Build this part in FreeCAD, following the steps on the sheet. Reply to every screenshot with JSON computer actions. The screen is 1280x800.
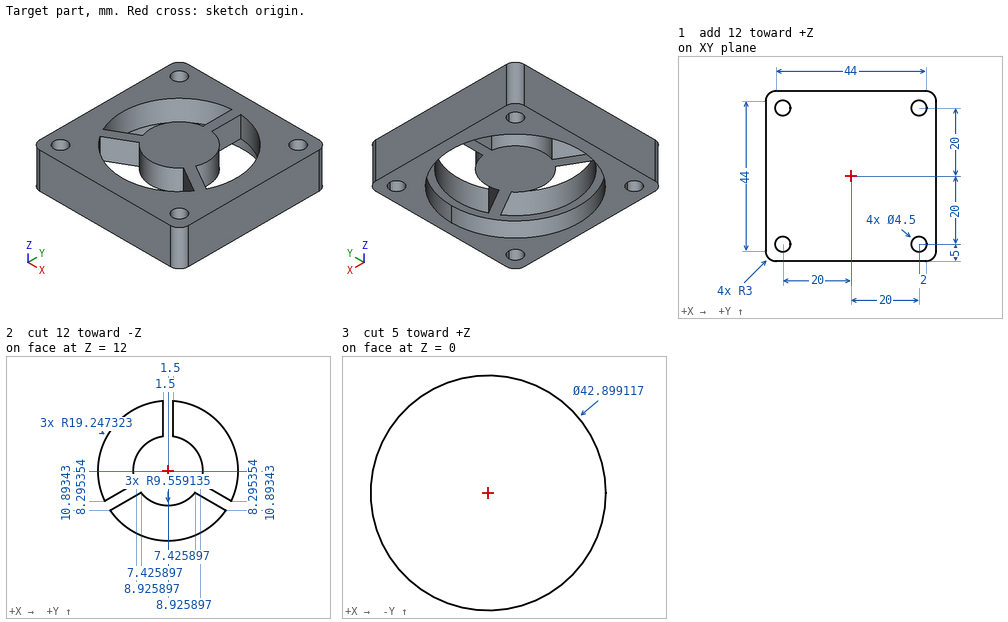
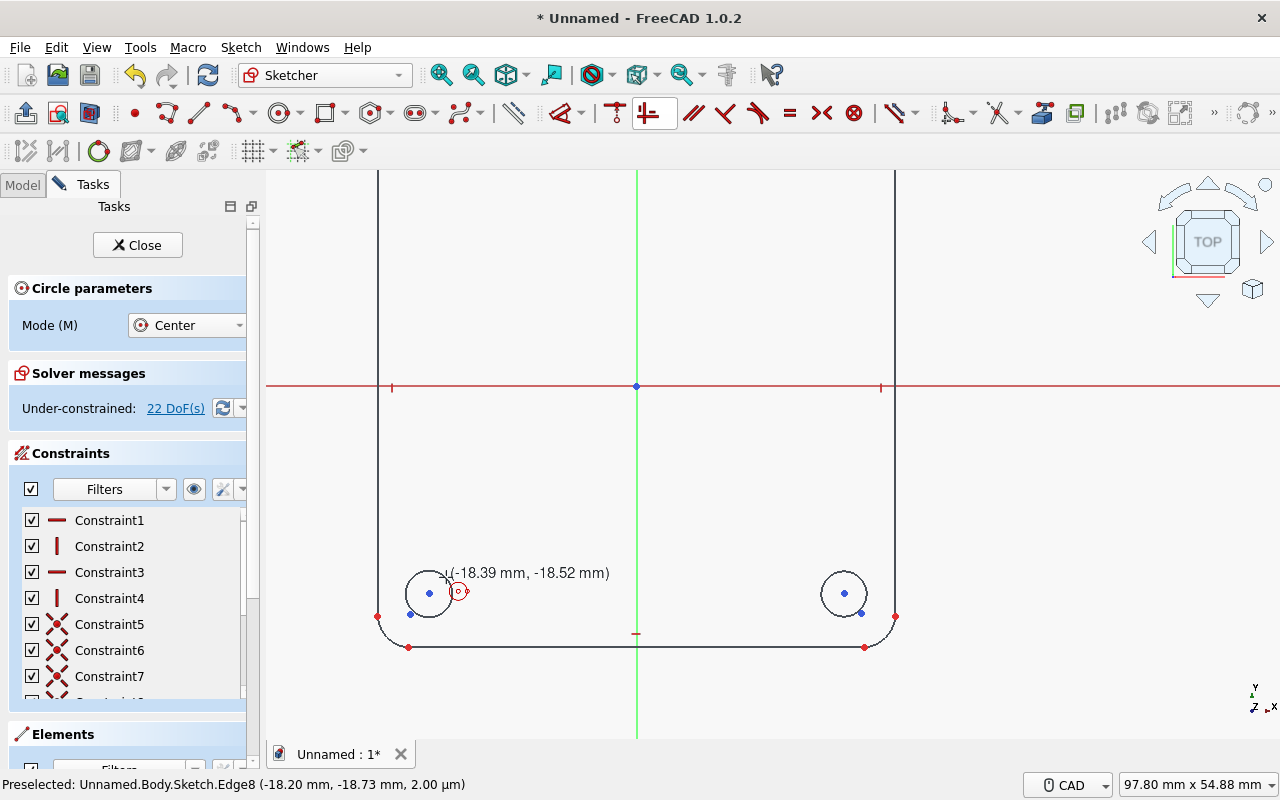
{"action": "scroll", "coordinate": [843, 594], "scroll_direction": "down", "scroll_amount": 2}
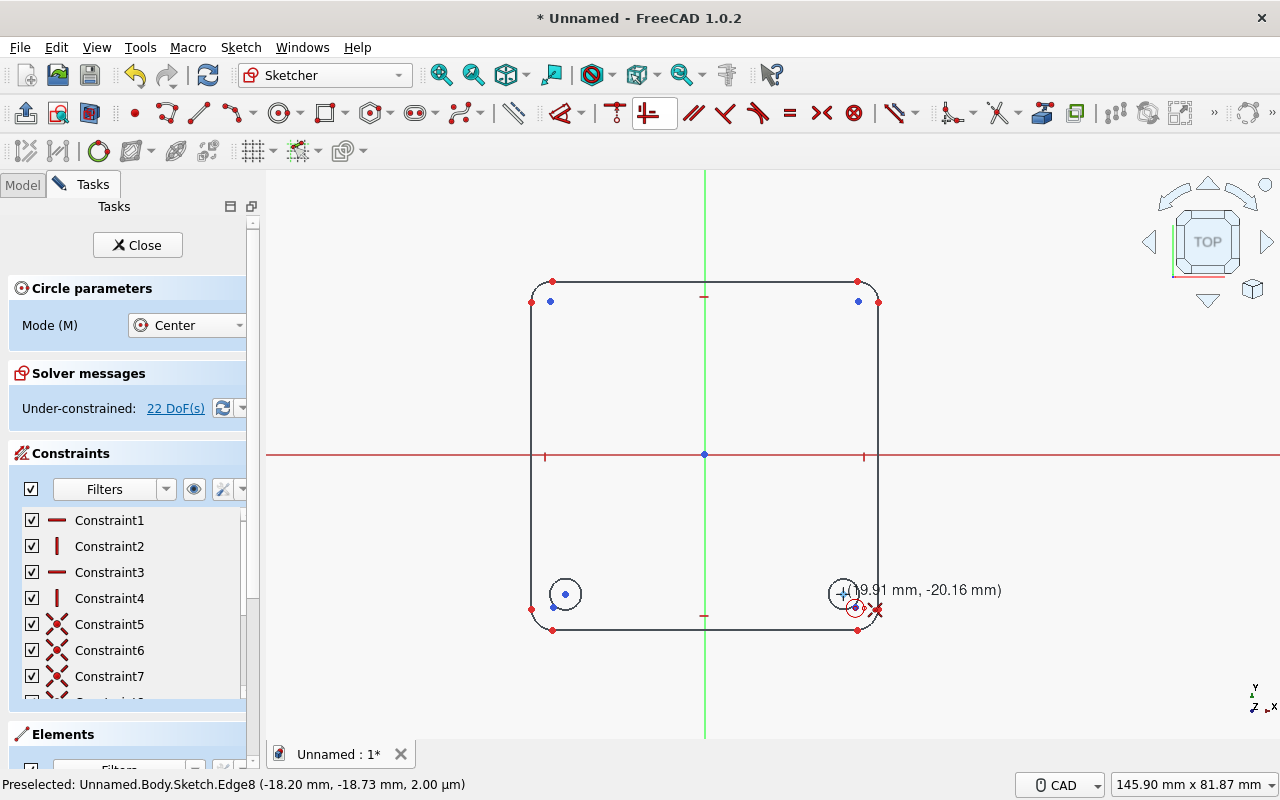
{"action": "scroll", "coordinate": [844, 316], "scroll_direction": "up", "scroll_amount": 2}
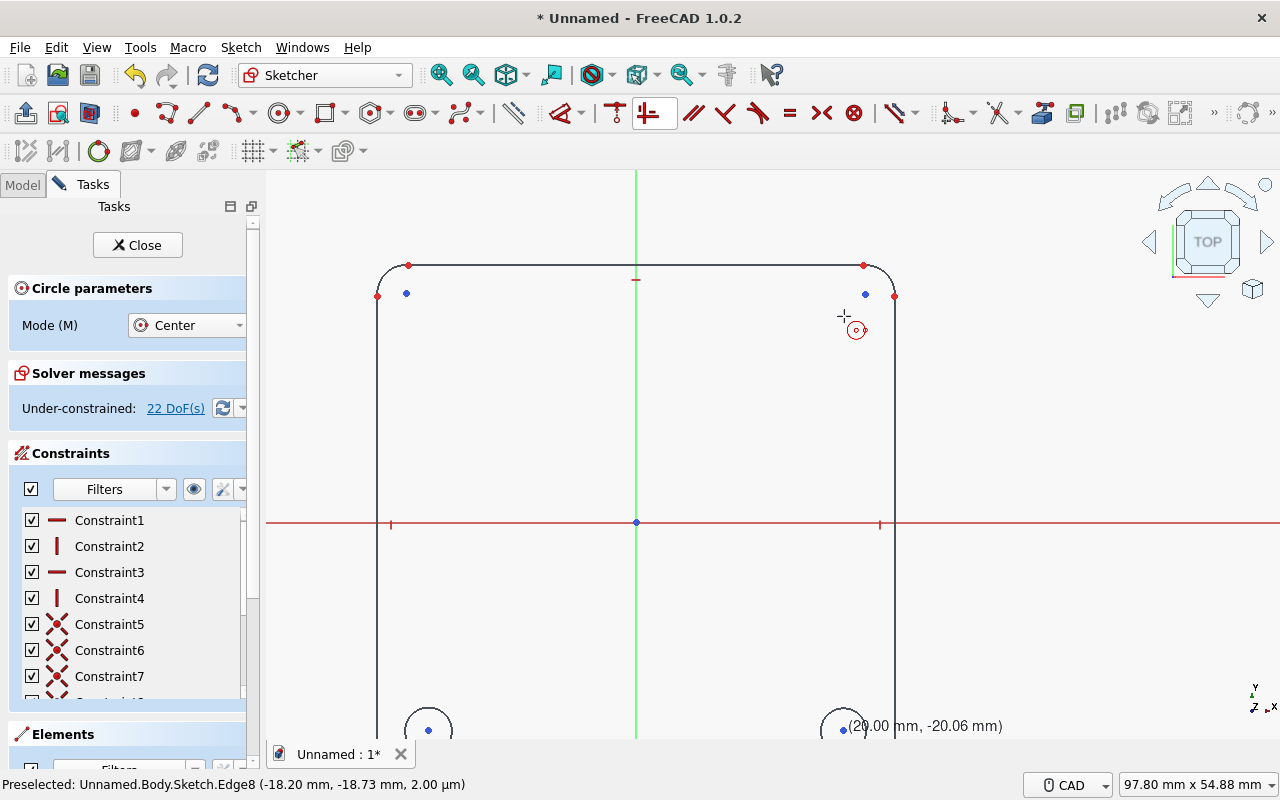
{"action": "left_click", "coordinate": [843, 316]}
{"action": "left_click", "coordinate": [827, 299]}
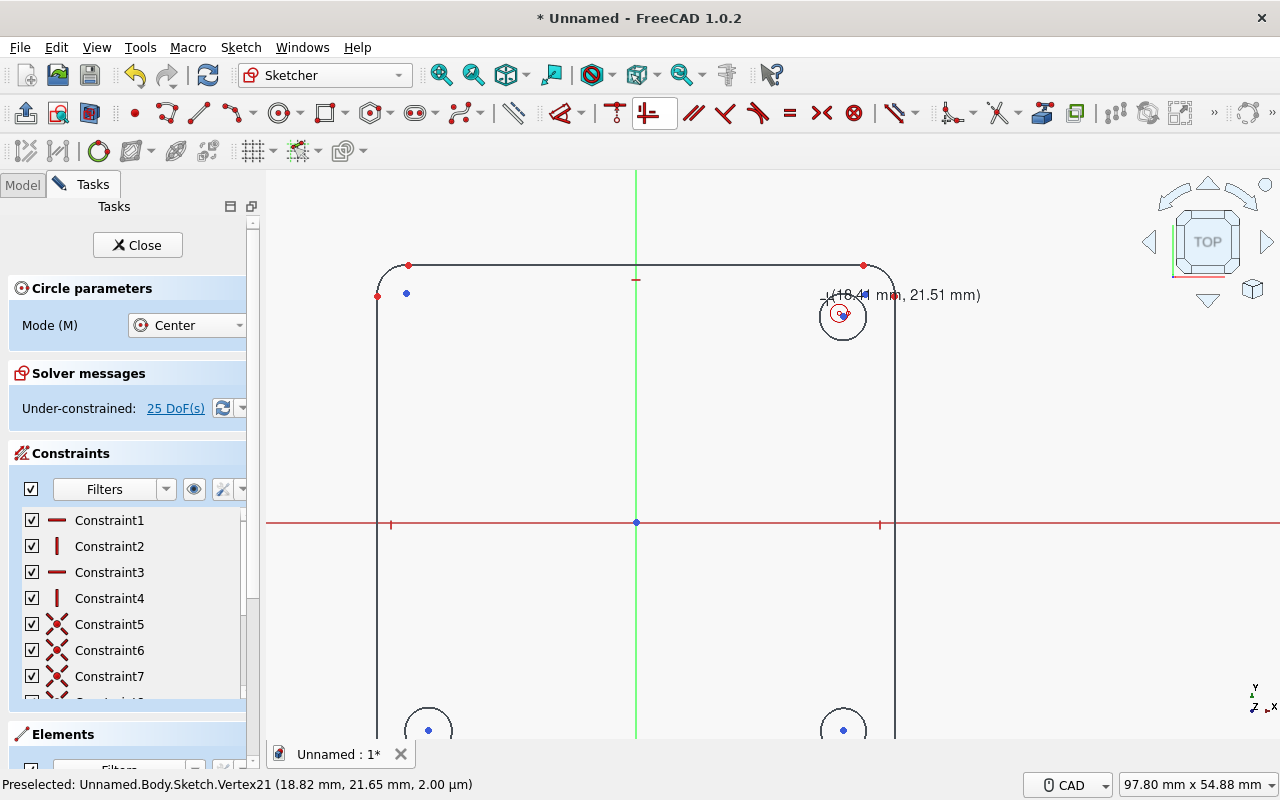
{"action": "left_click", "coordinate": [429, 316]}
{"action": "left_click", "coordinate": [445, 299]}
{"action": "key", "text": "Escape"}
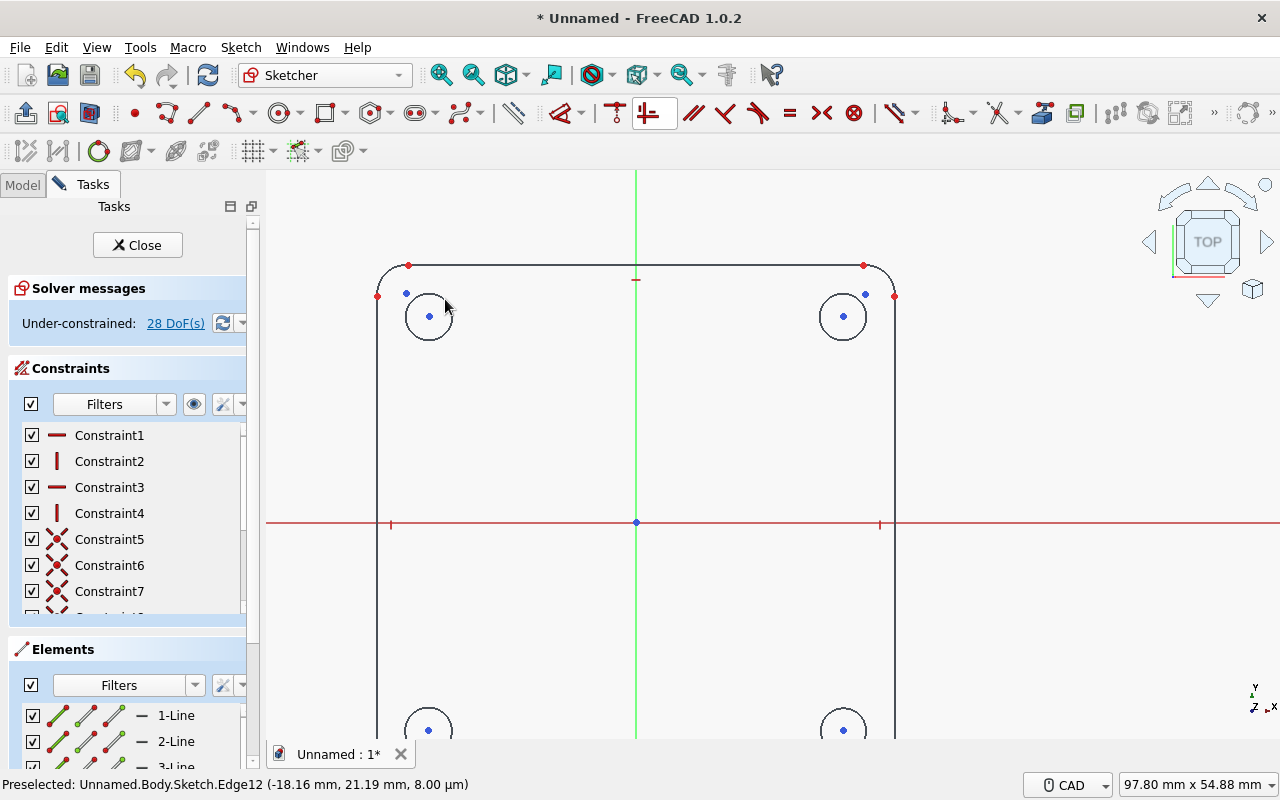
{"action": "left_click", "coordinate": [727, 265]}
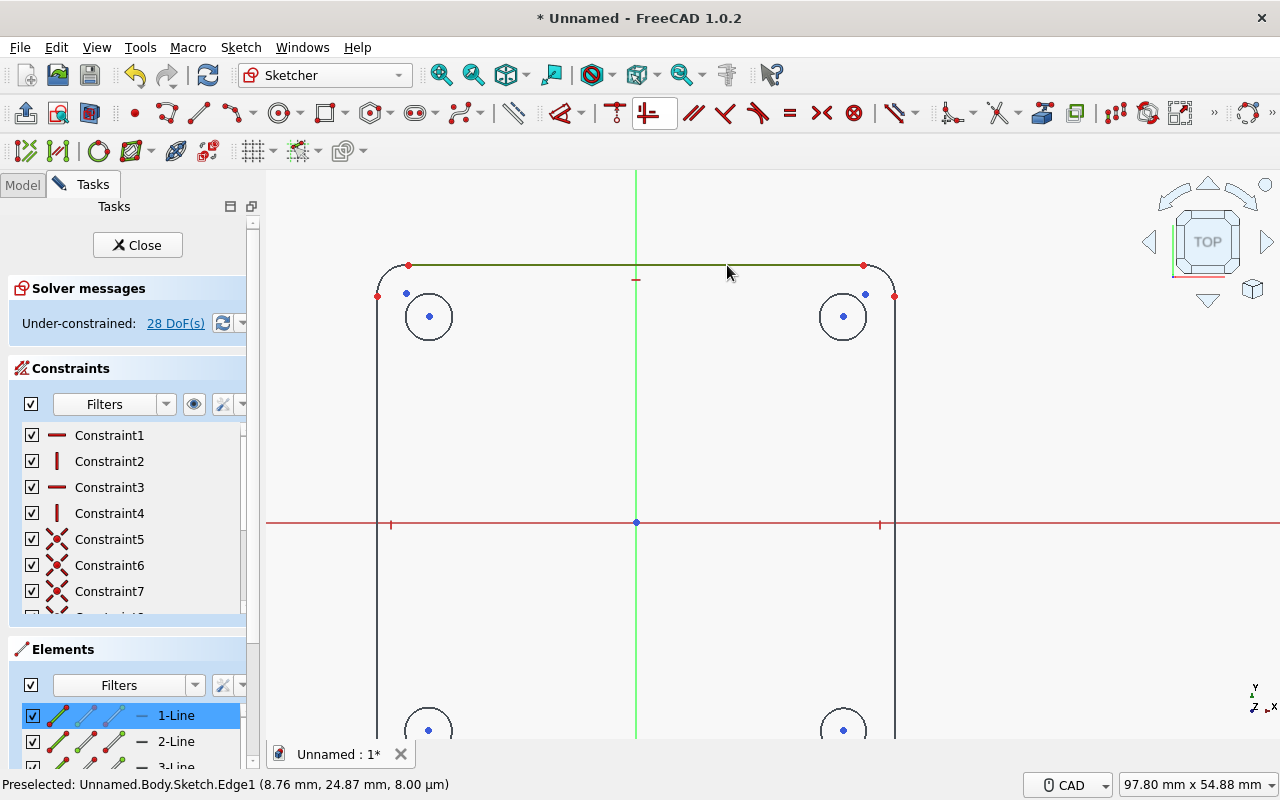
{"action": "left_click", "coordinate": [394, 268]}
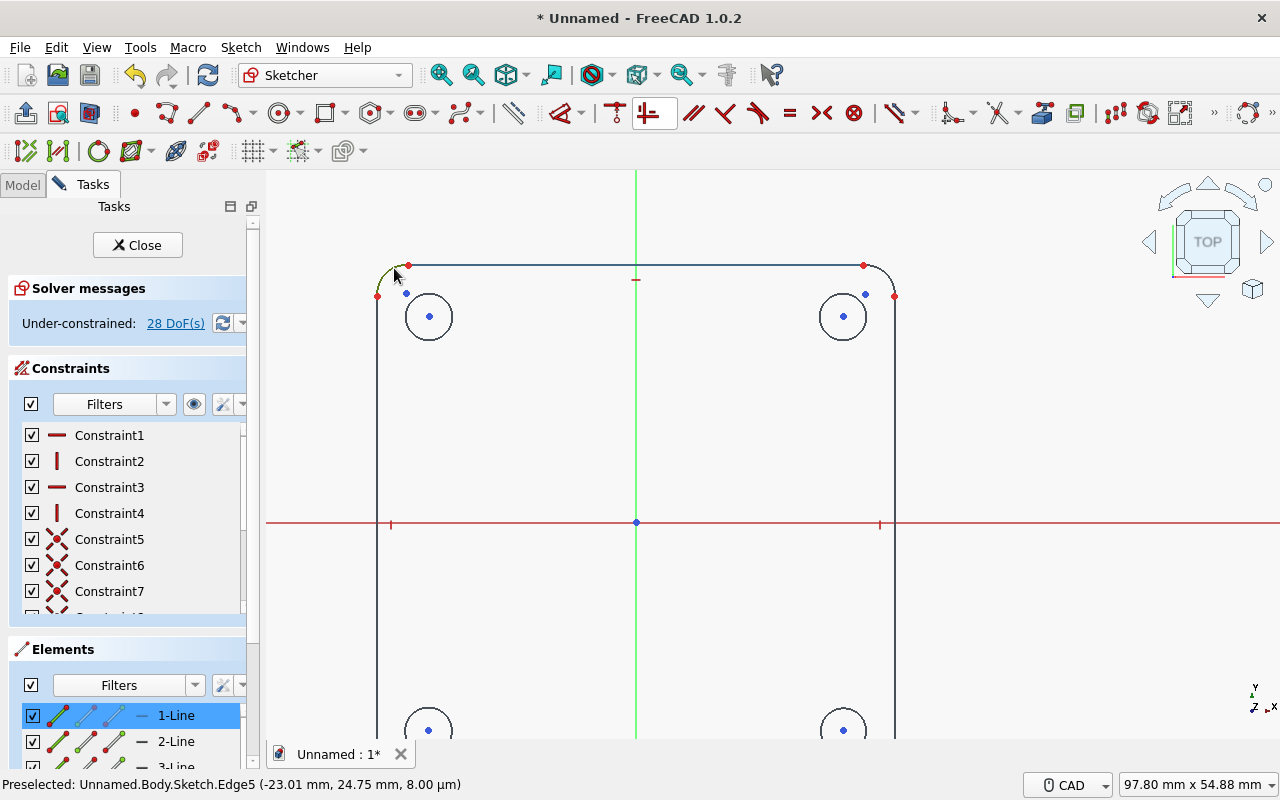
{"action": "left_click", "coordinate": [758, 114]}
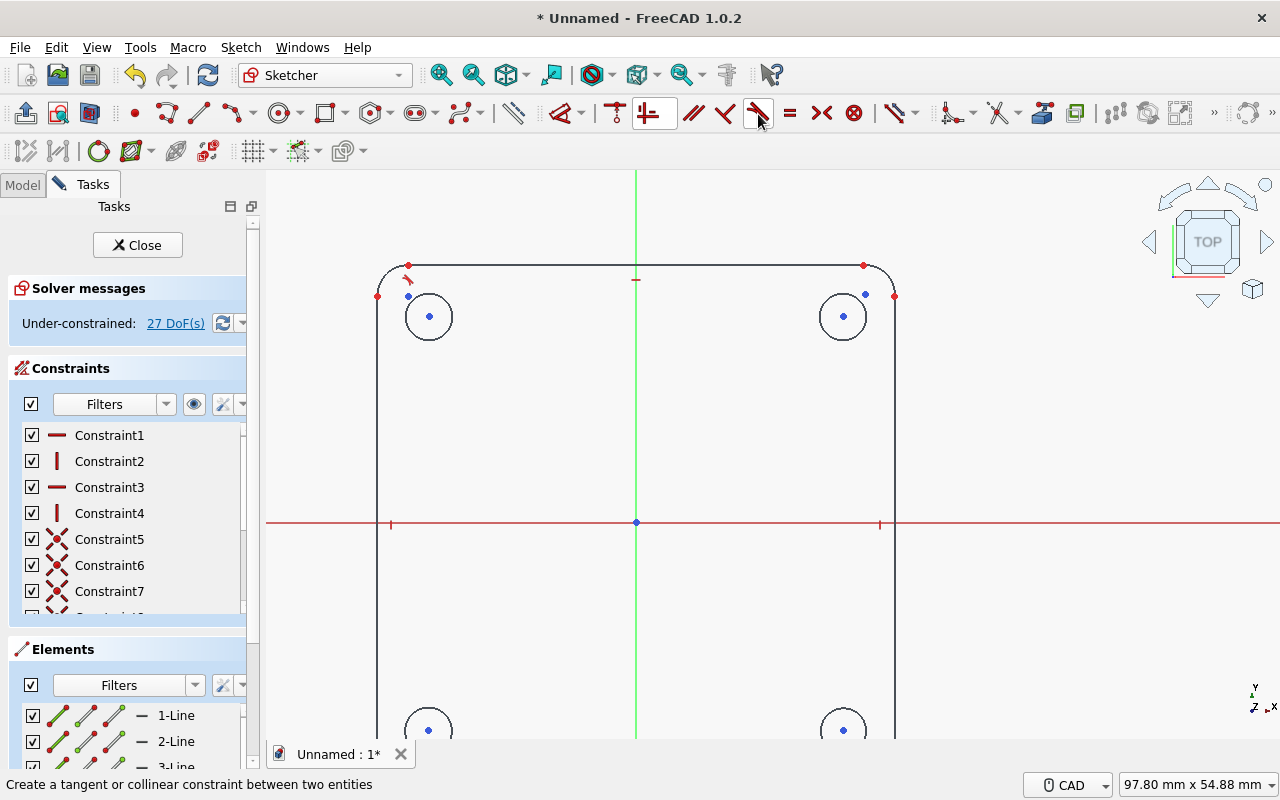
{"action": "left_click", "coordinate": [727, 265]}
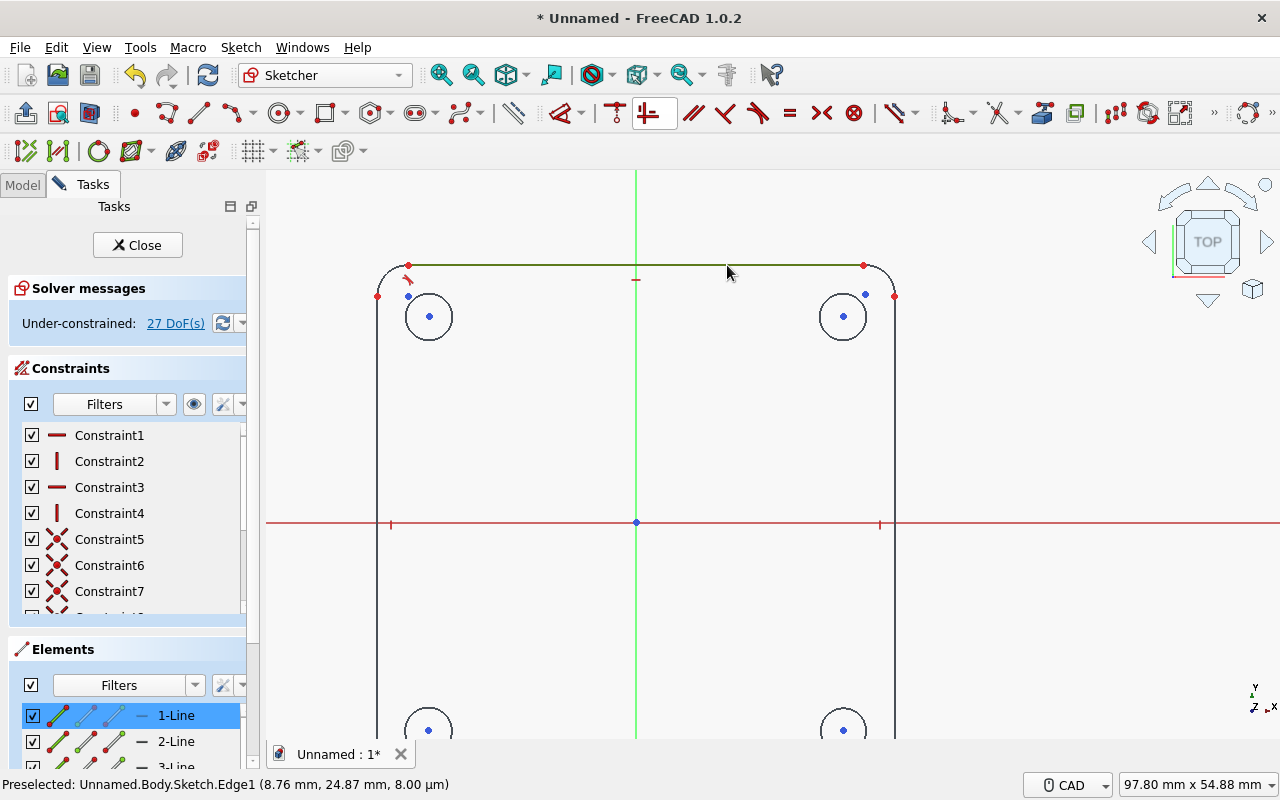
{"action": "left_click", "coordinate": [892, 282]}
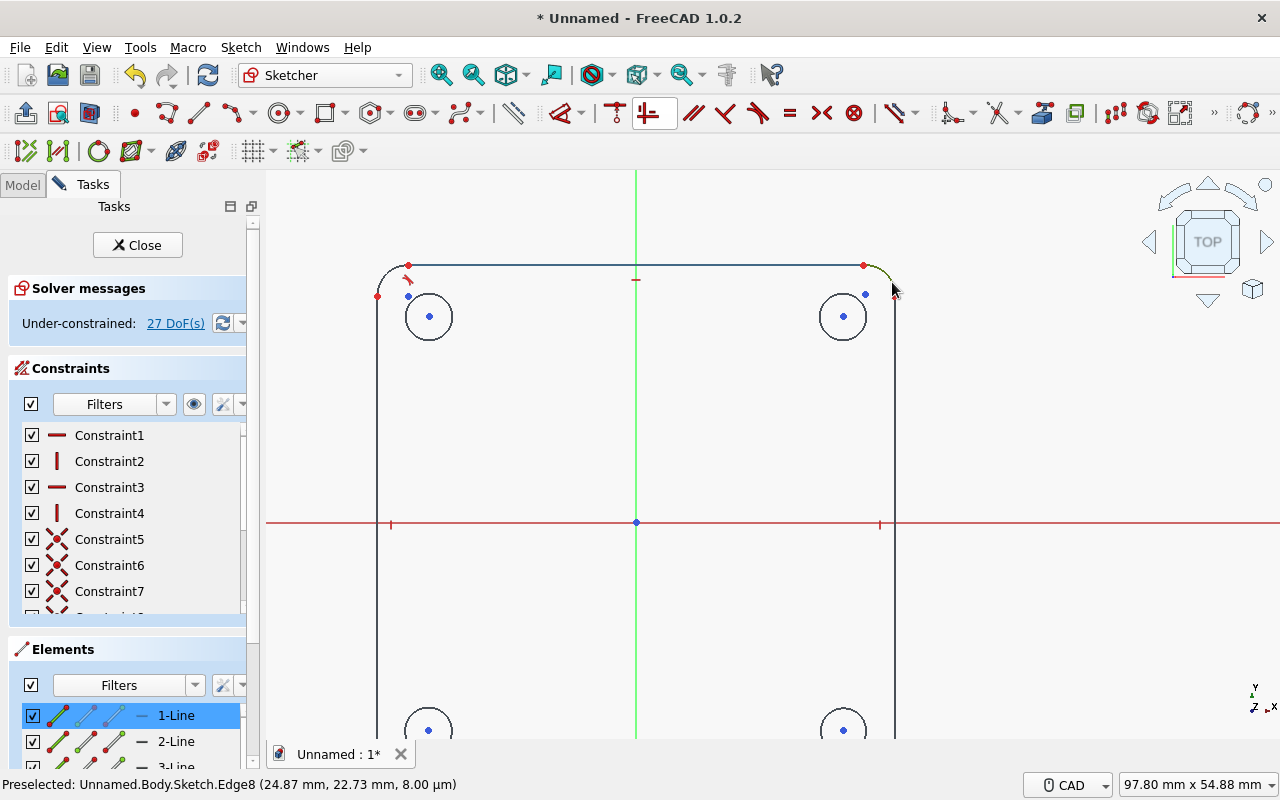
{"action": "left_click", "coordinate": [758, 114]}